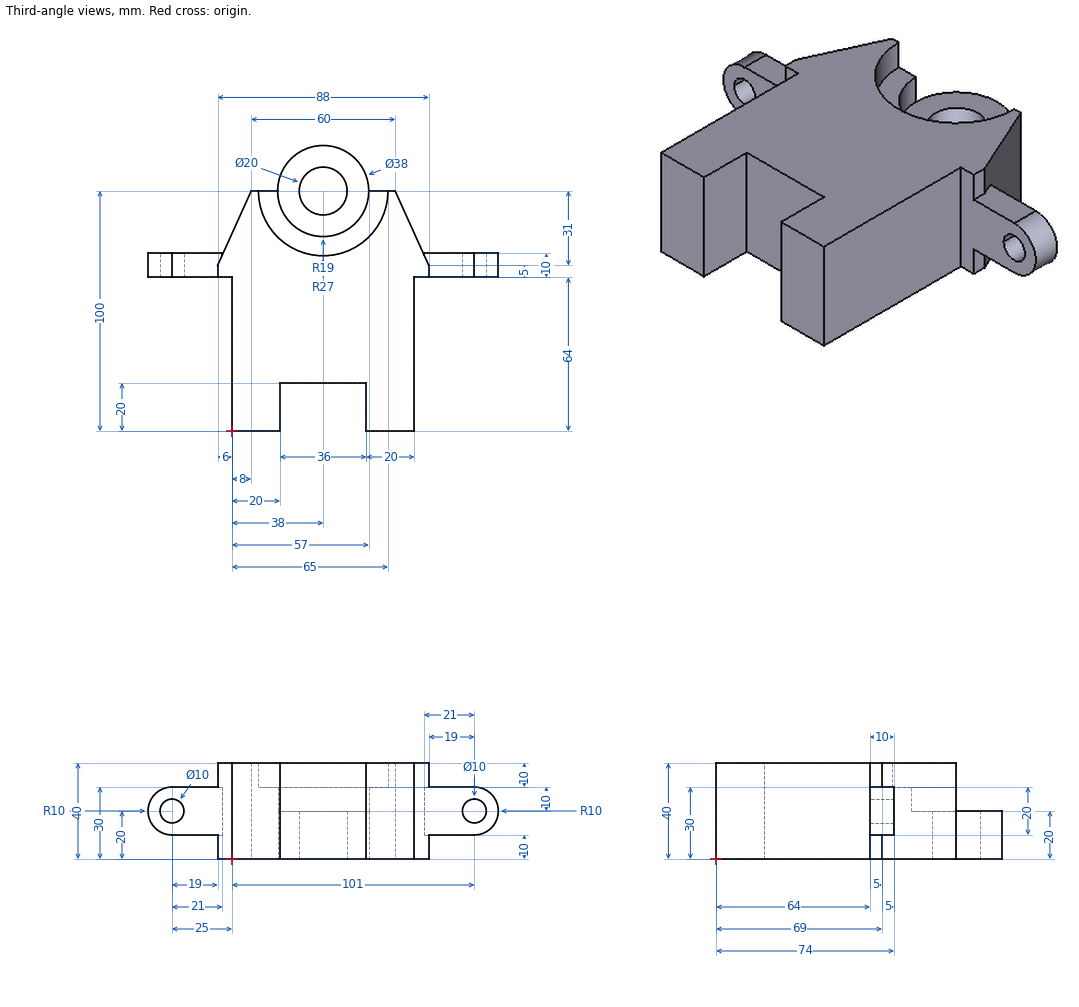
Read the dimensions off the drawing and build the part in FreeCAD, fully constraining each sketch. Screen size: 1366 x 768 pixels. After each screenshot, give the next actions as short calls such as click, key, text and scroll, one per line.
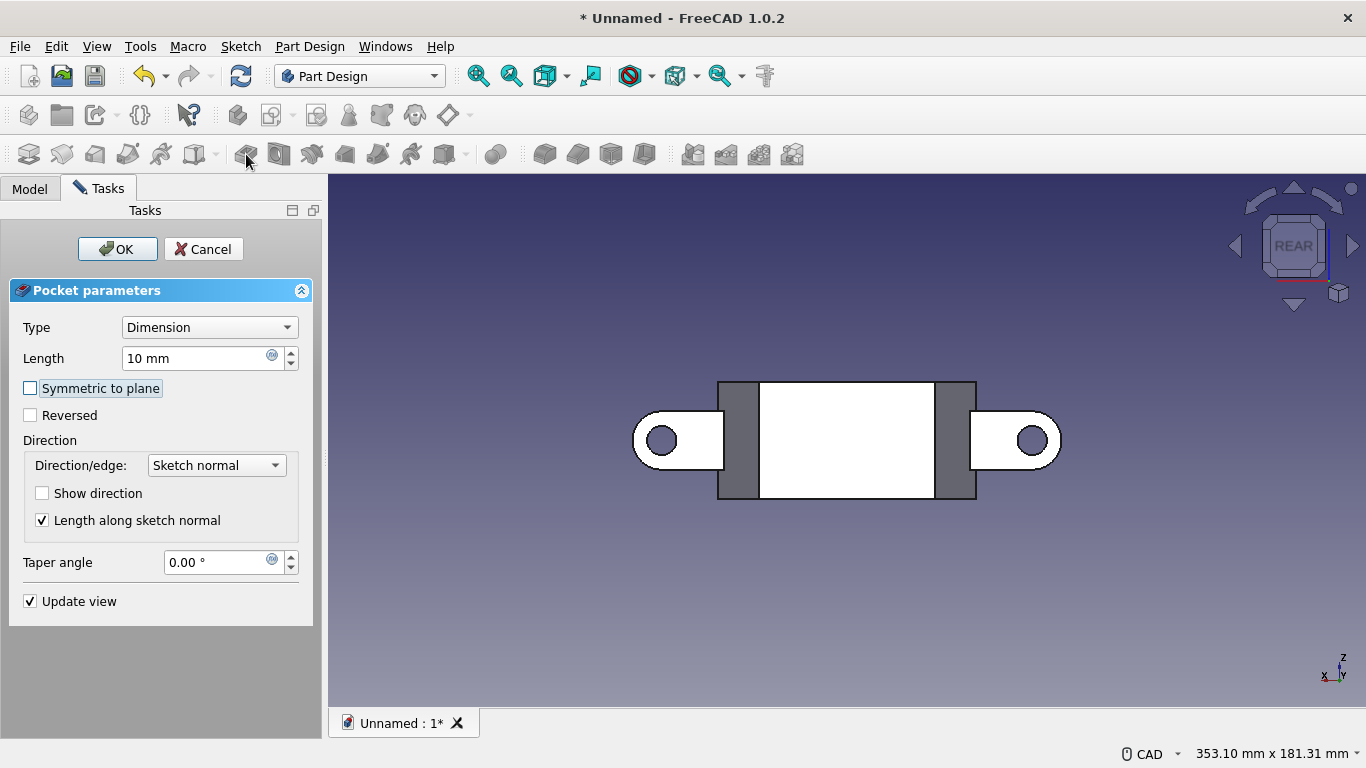
click(118, 249)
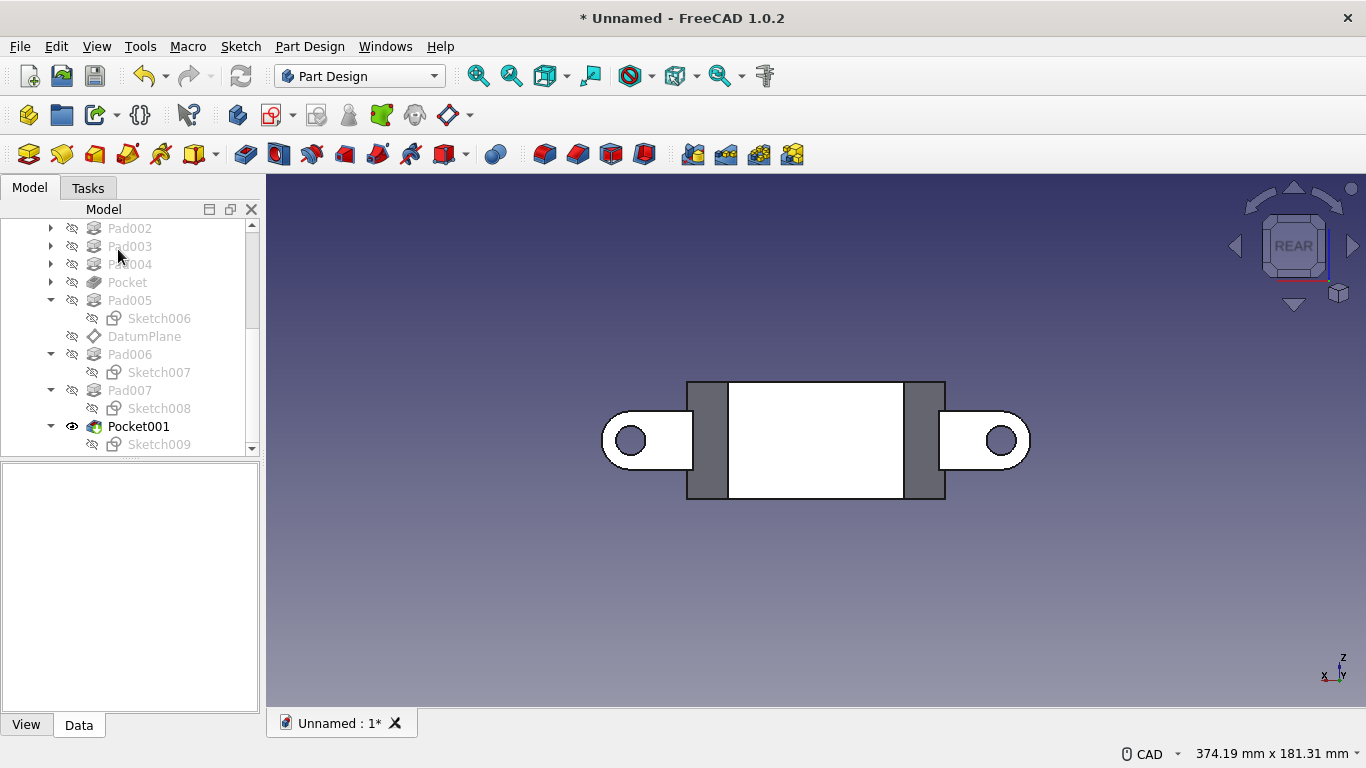
click(479, 76)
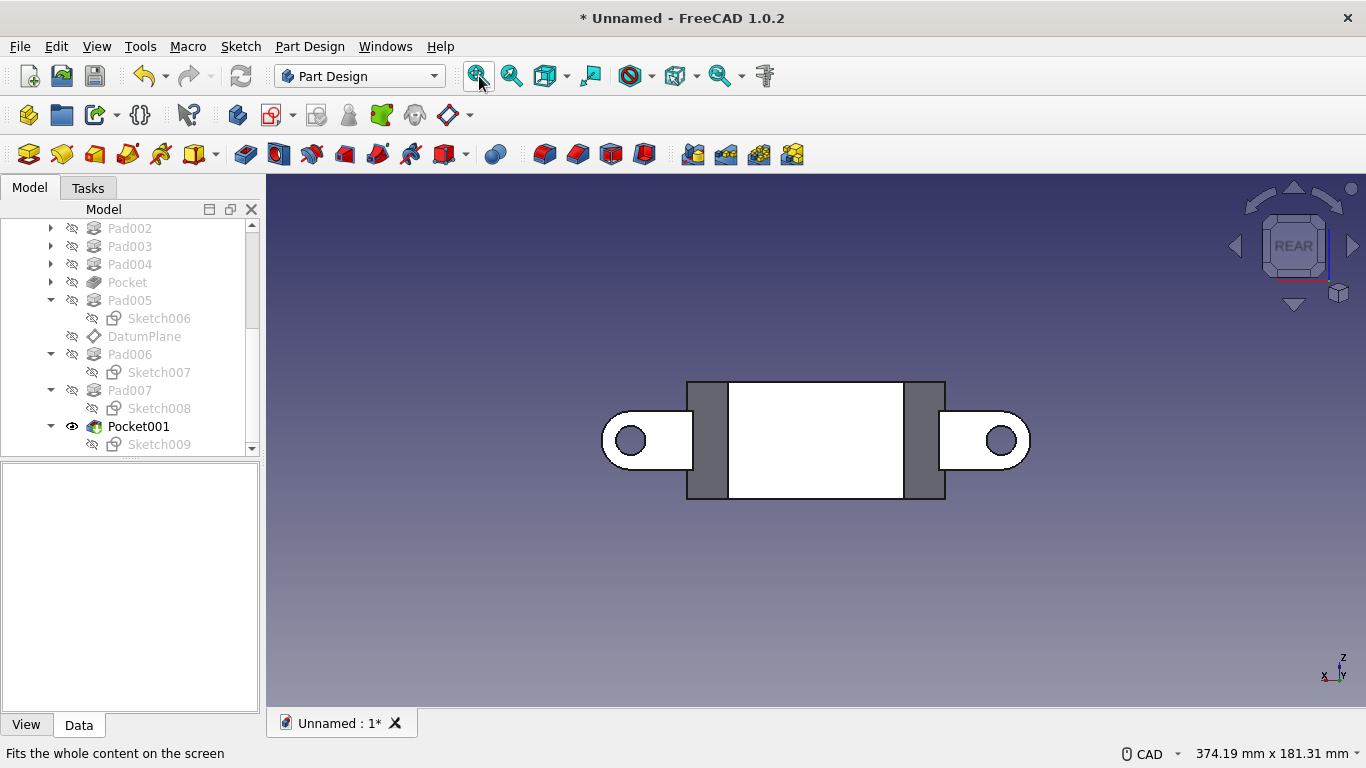
key(0)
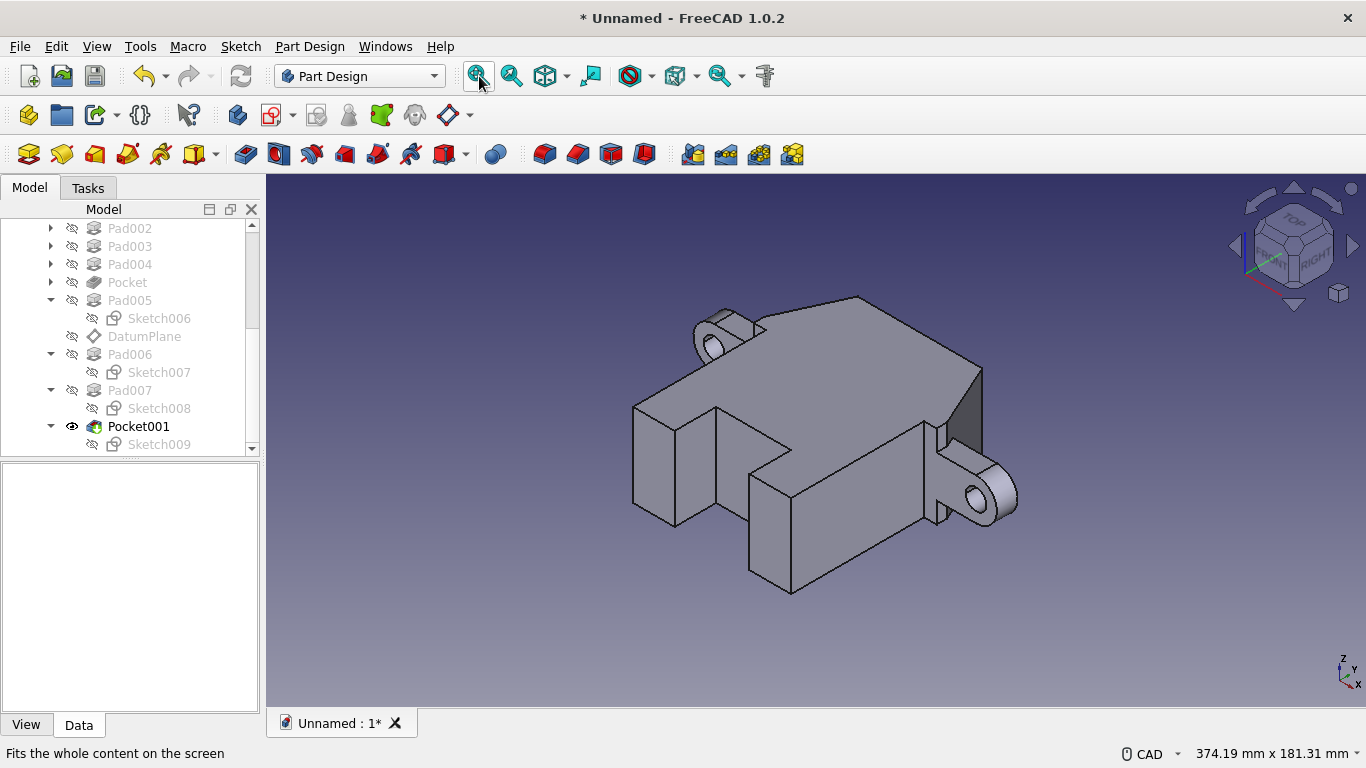
click(846, 374)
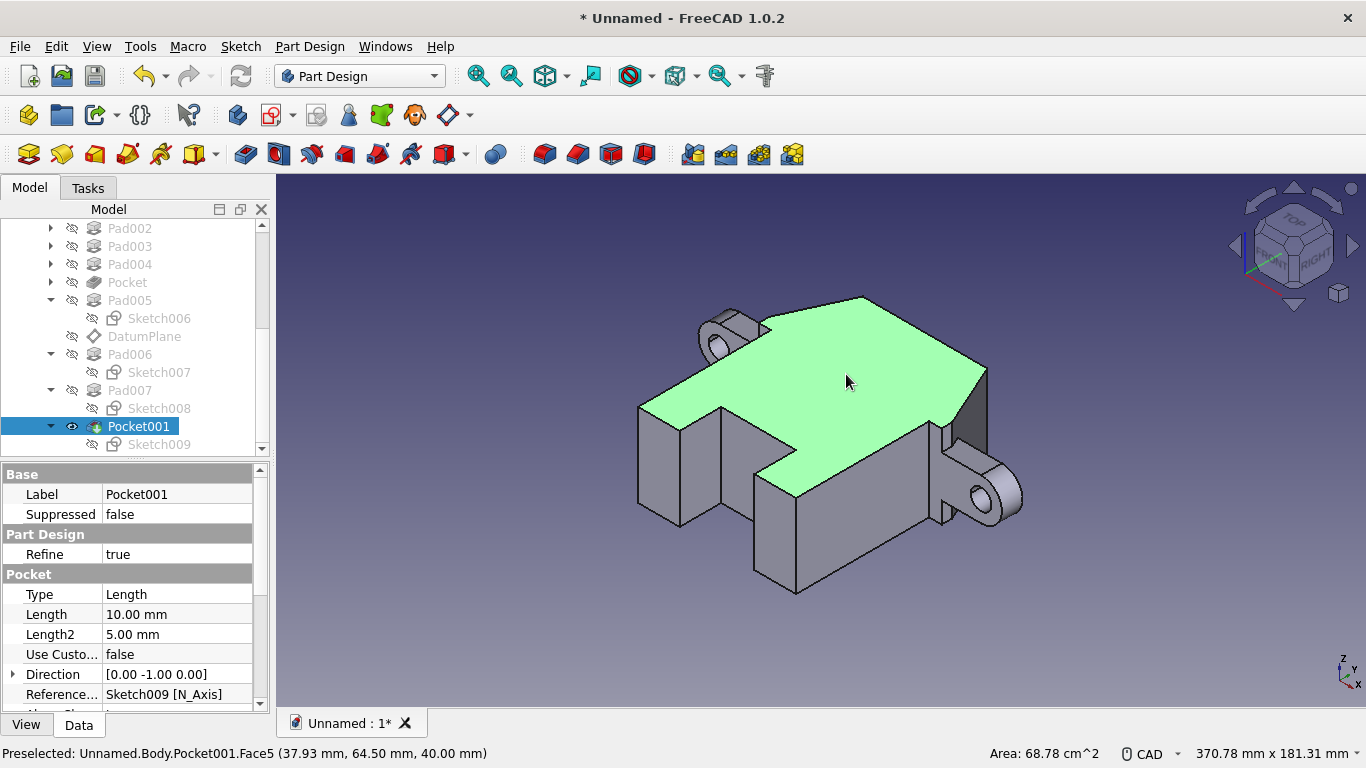
click(270, 116)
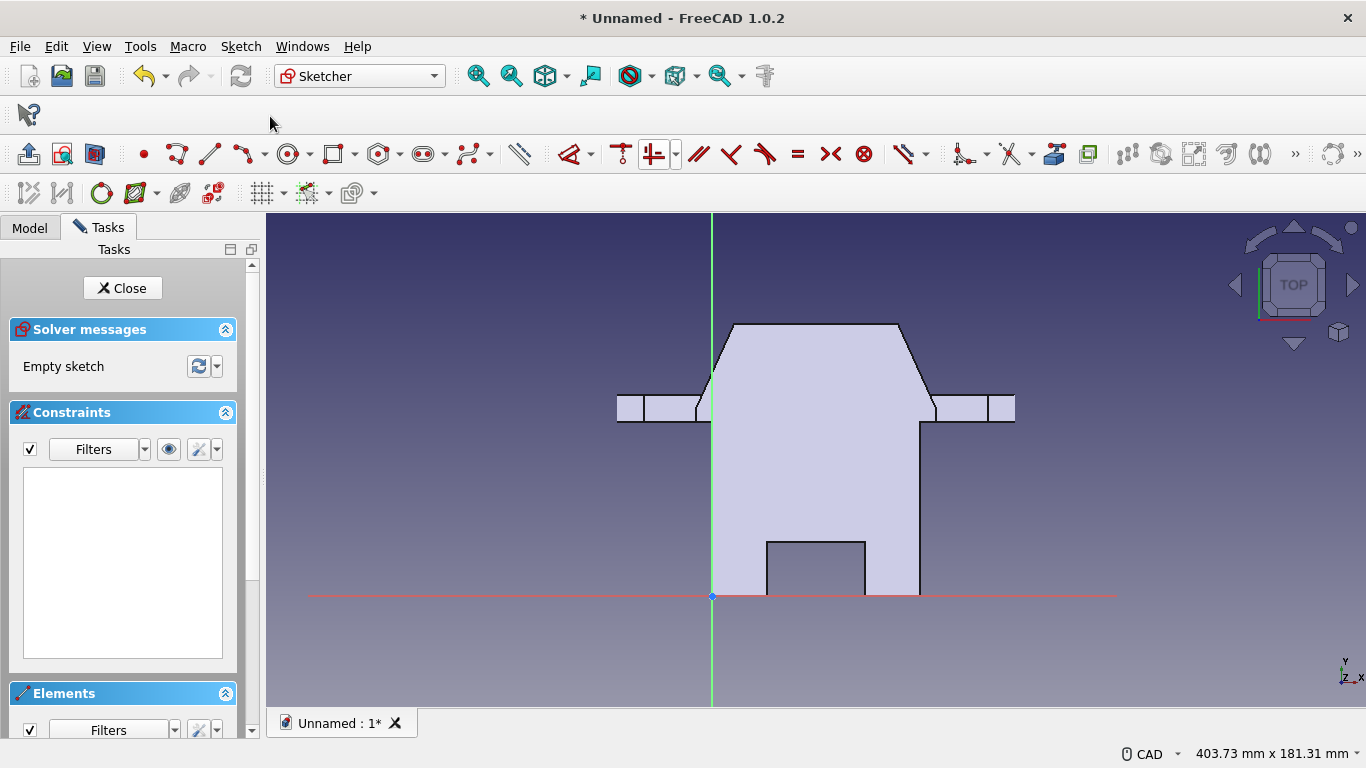
click(210, 154)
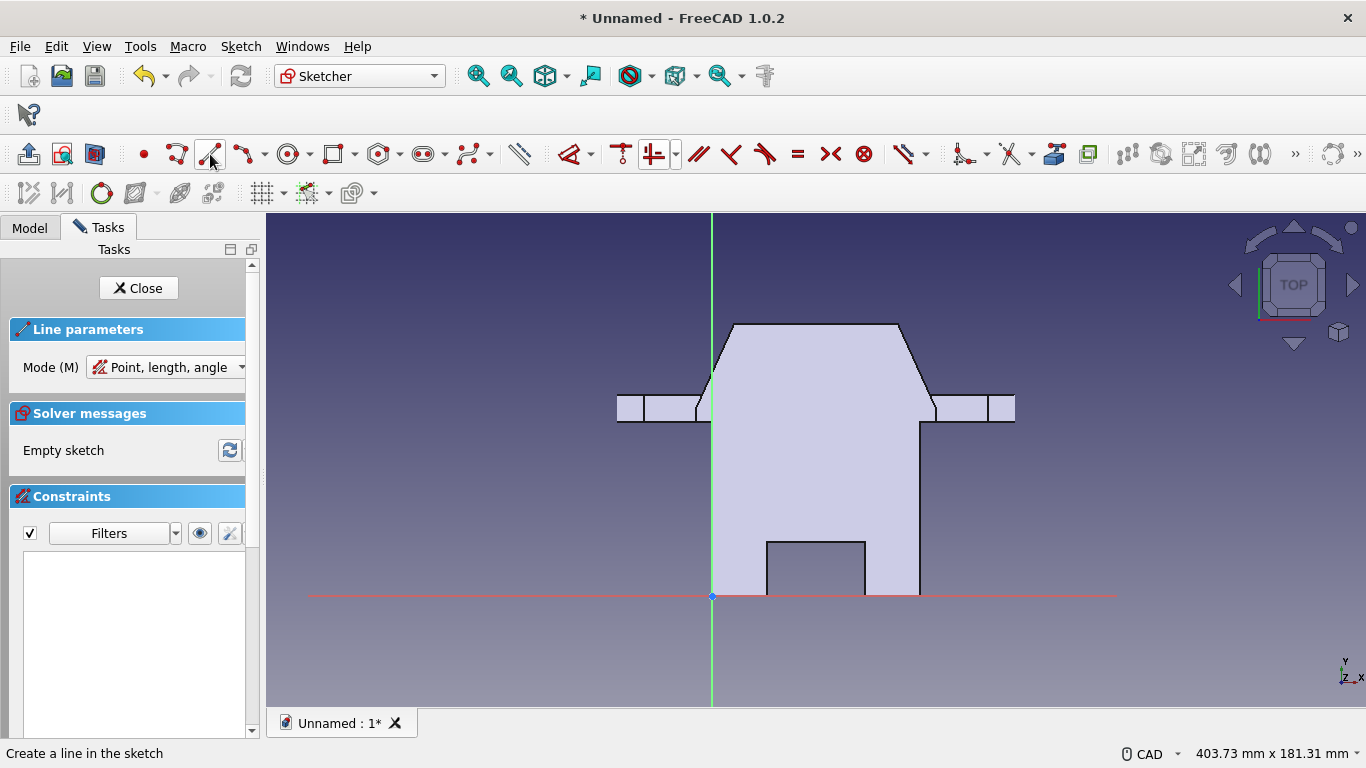
click(890, 324)
click(742, 324)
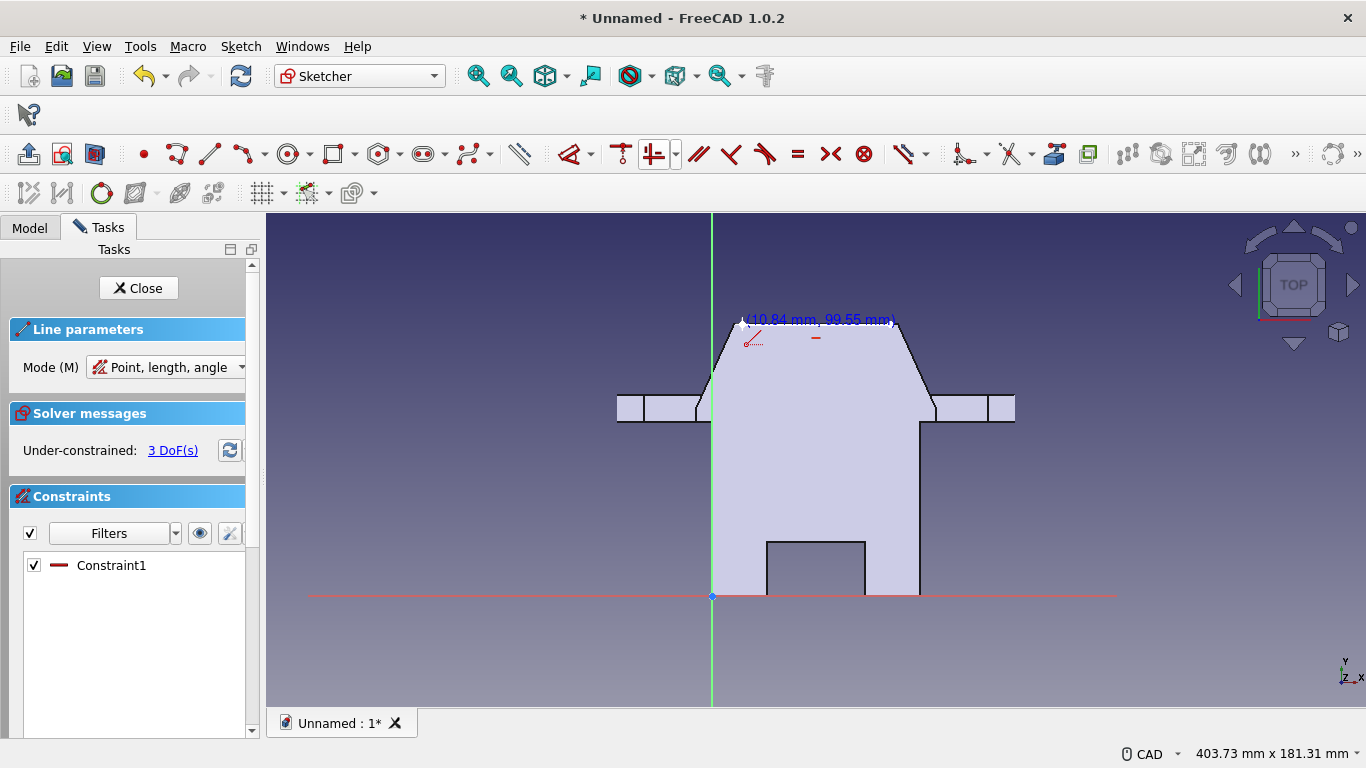
click(242, 154)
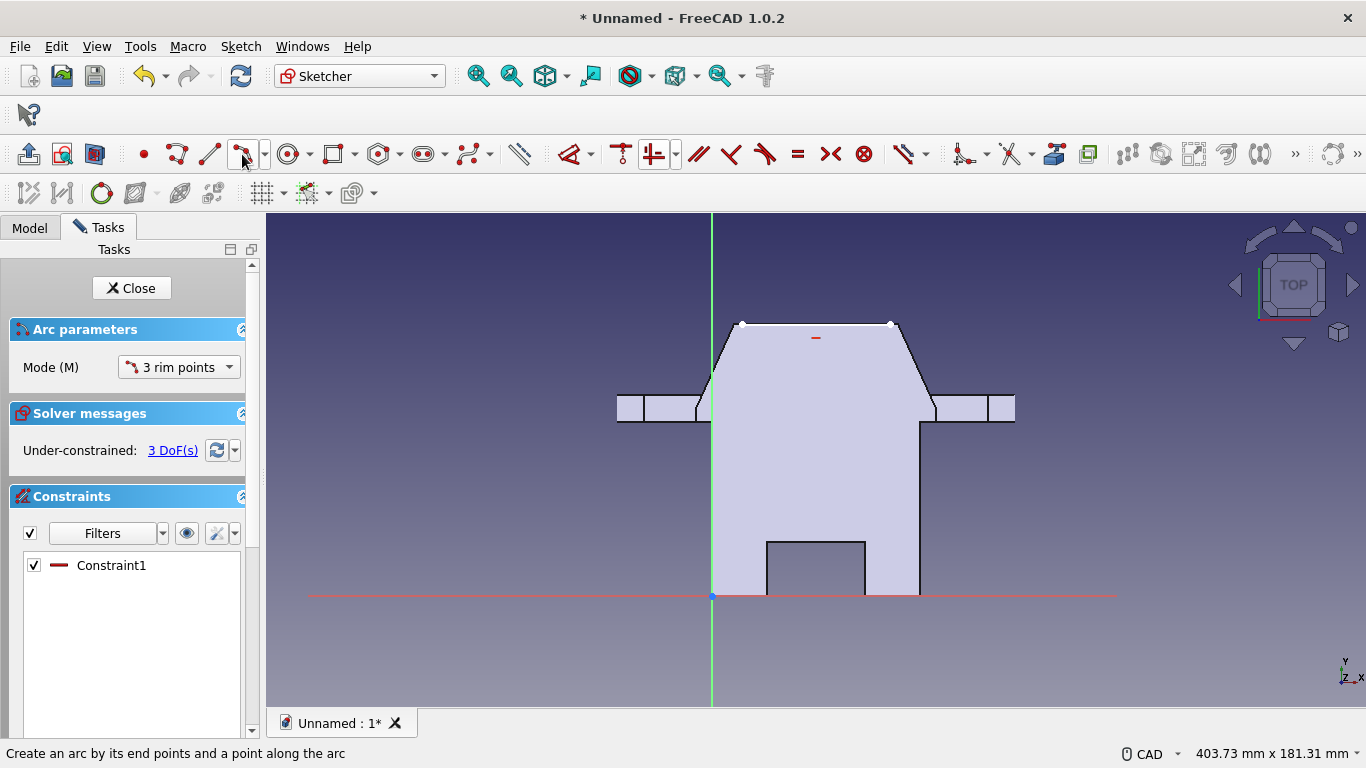
click(742, 325)
click(890, 325)
click(816, 397)
key(Escape)